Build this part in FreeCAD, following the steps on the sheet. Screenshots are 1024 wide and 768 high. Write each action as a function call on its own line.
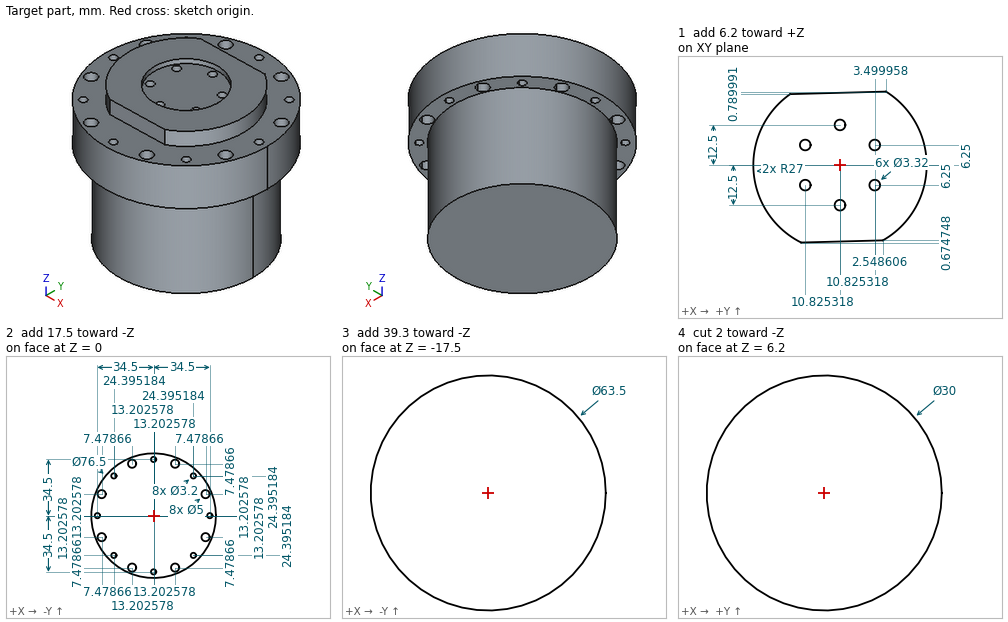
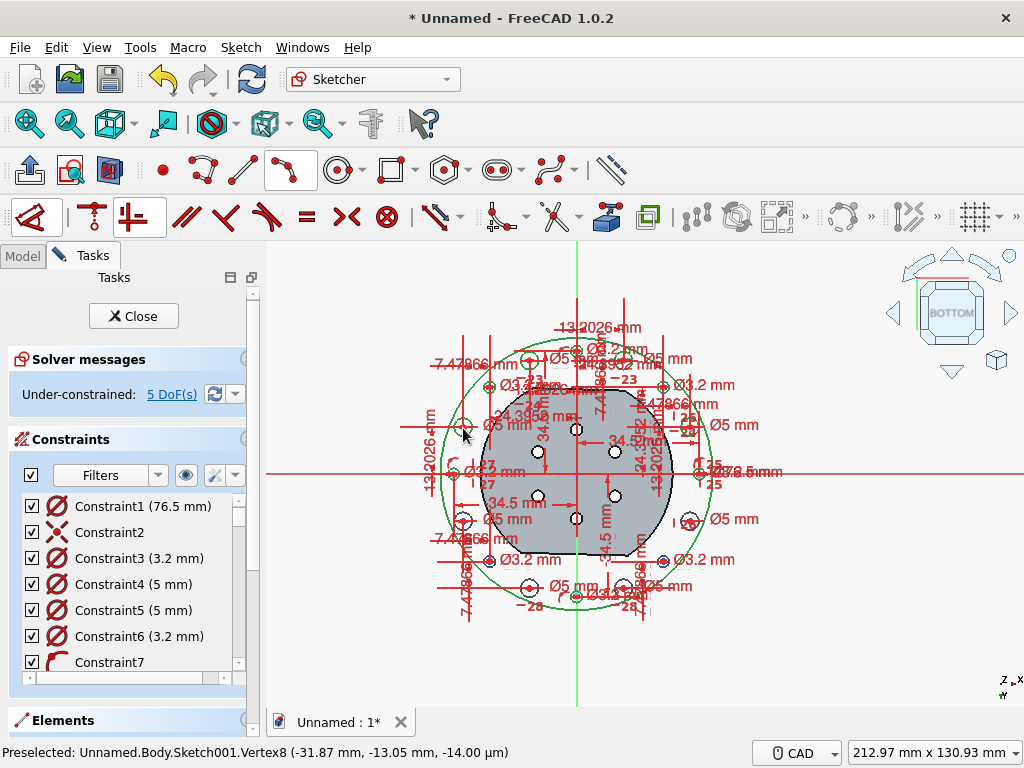
scroll(690, 521, up, 4)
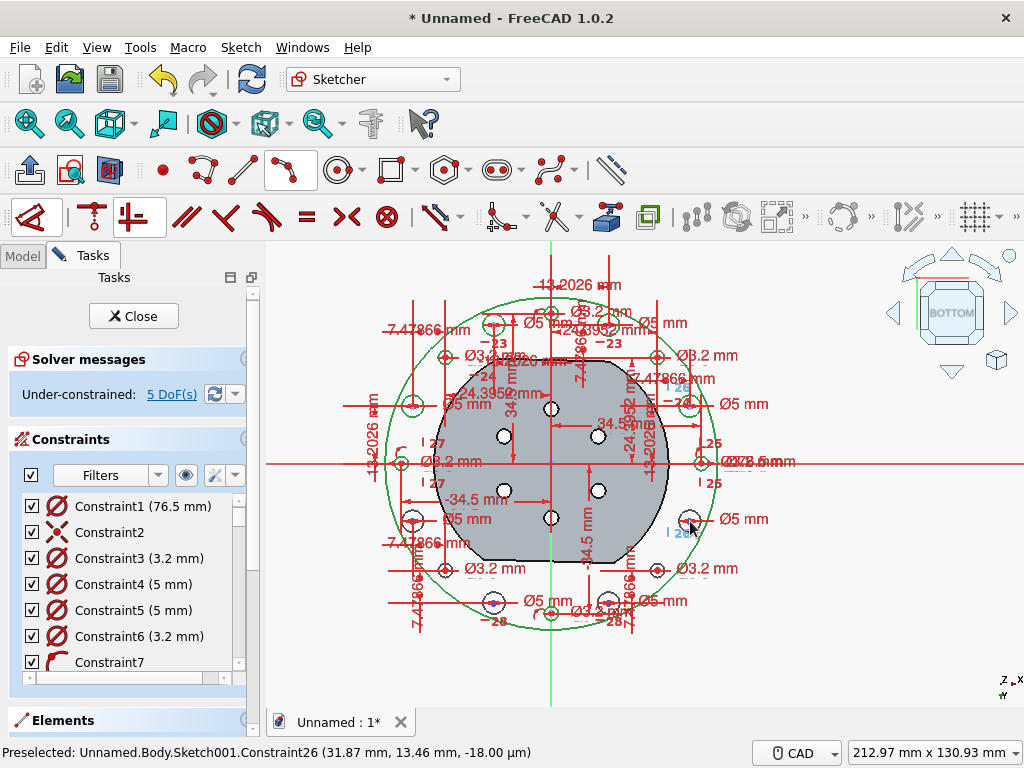
click(689, 521)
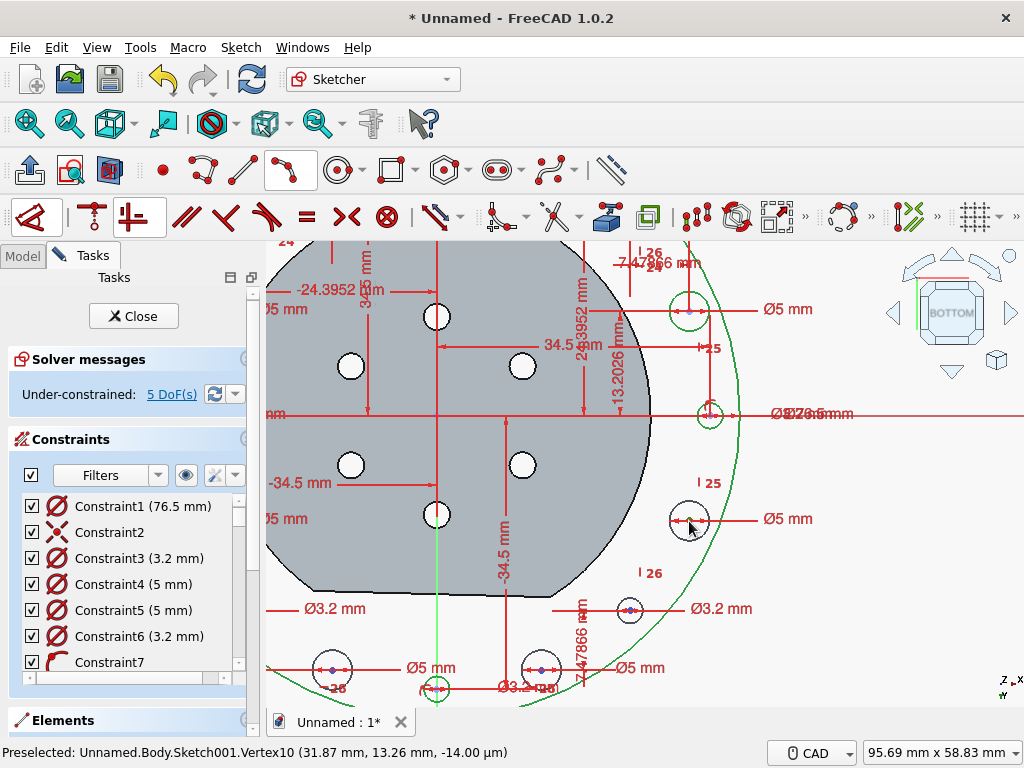
click(56, 218)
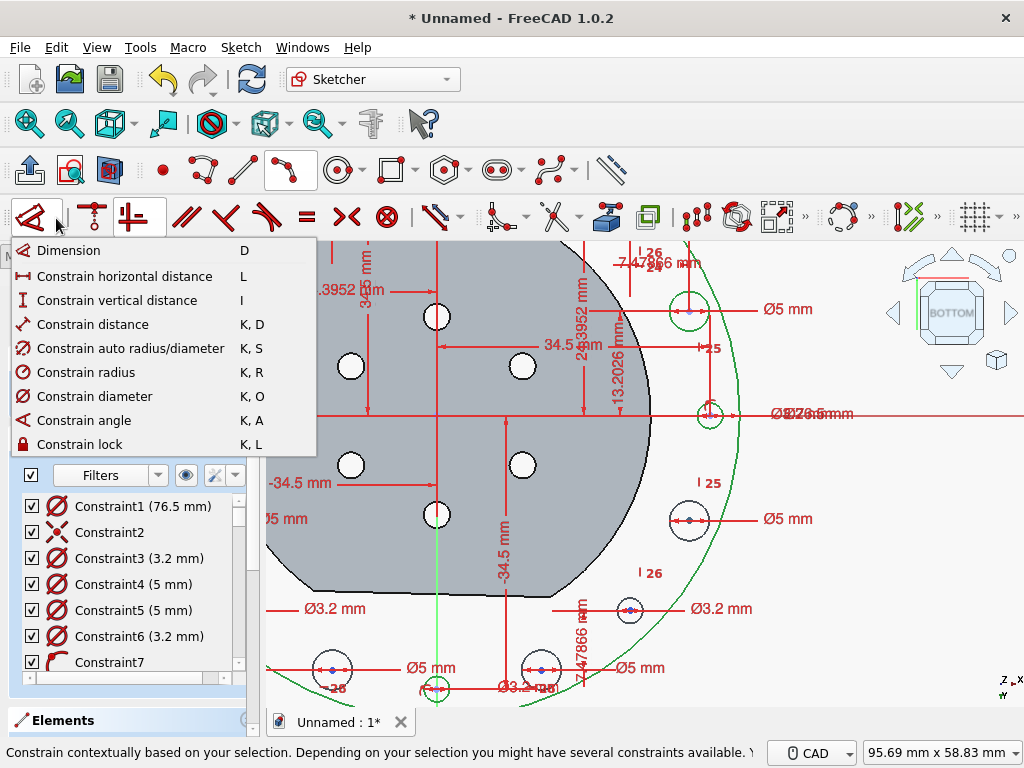
click(164, 300)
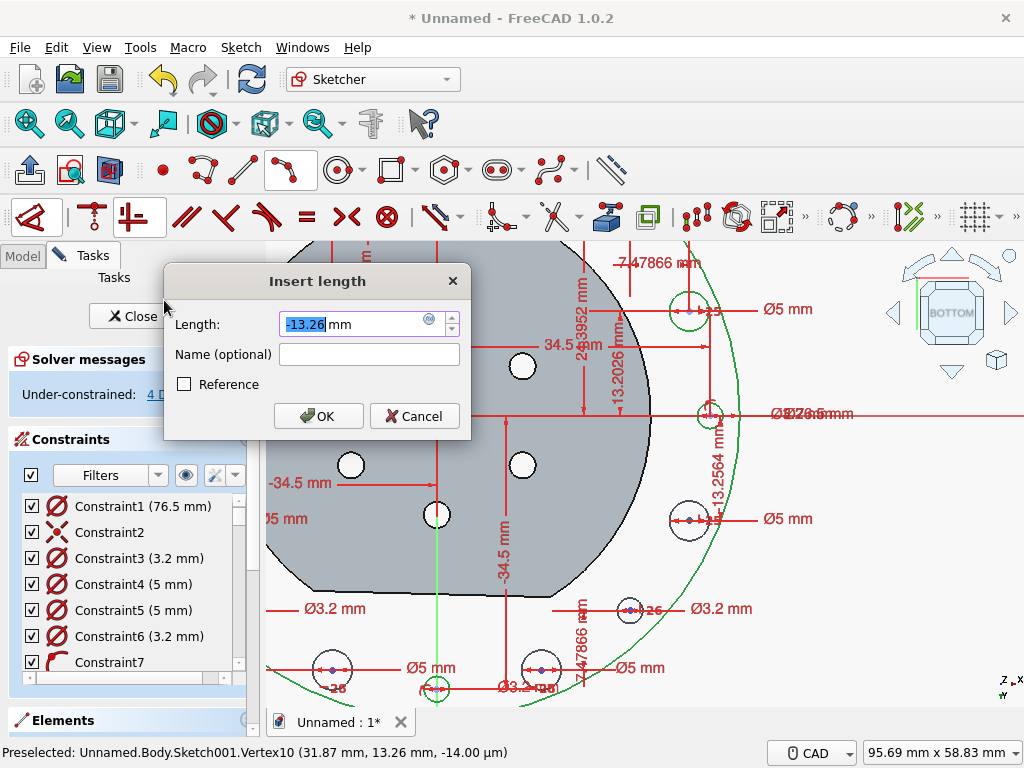
text(-13.202578)
key(Return)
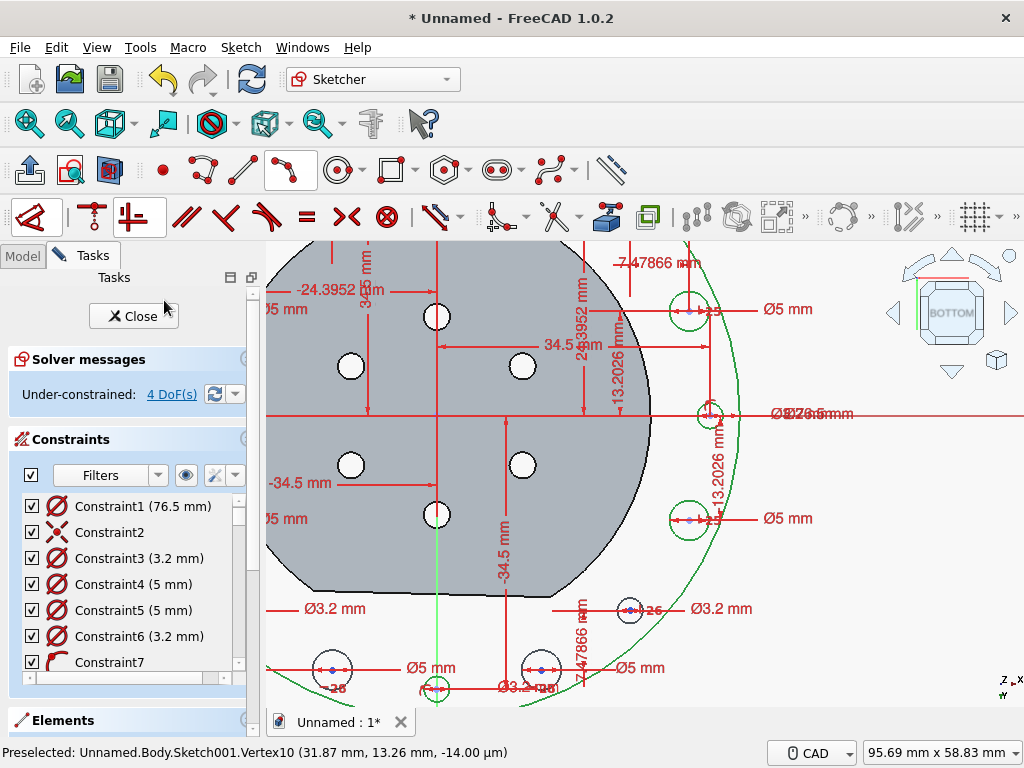
click(630, 611)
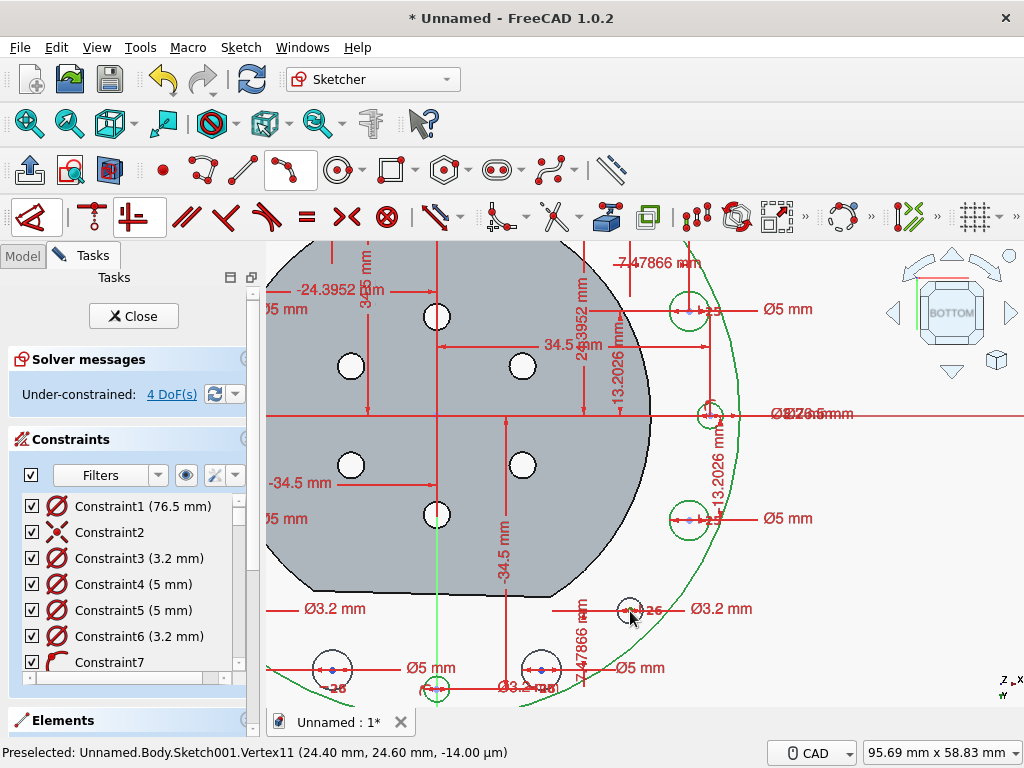
click(56, 218)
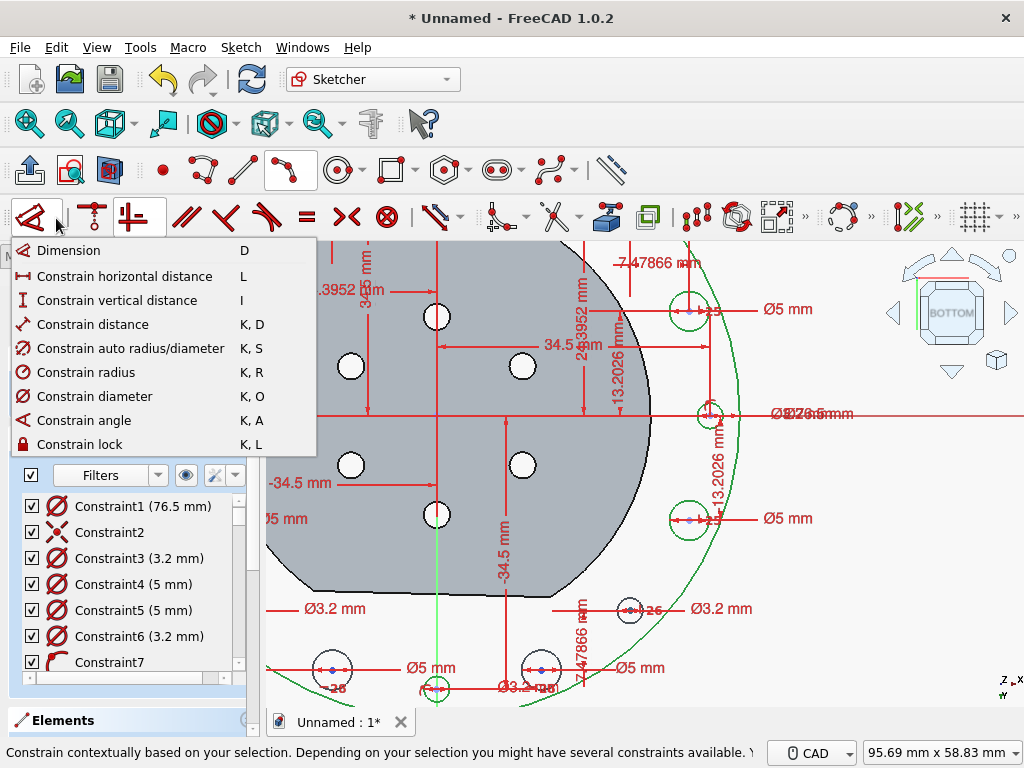
click(164, 300)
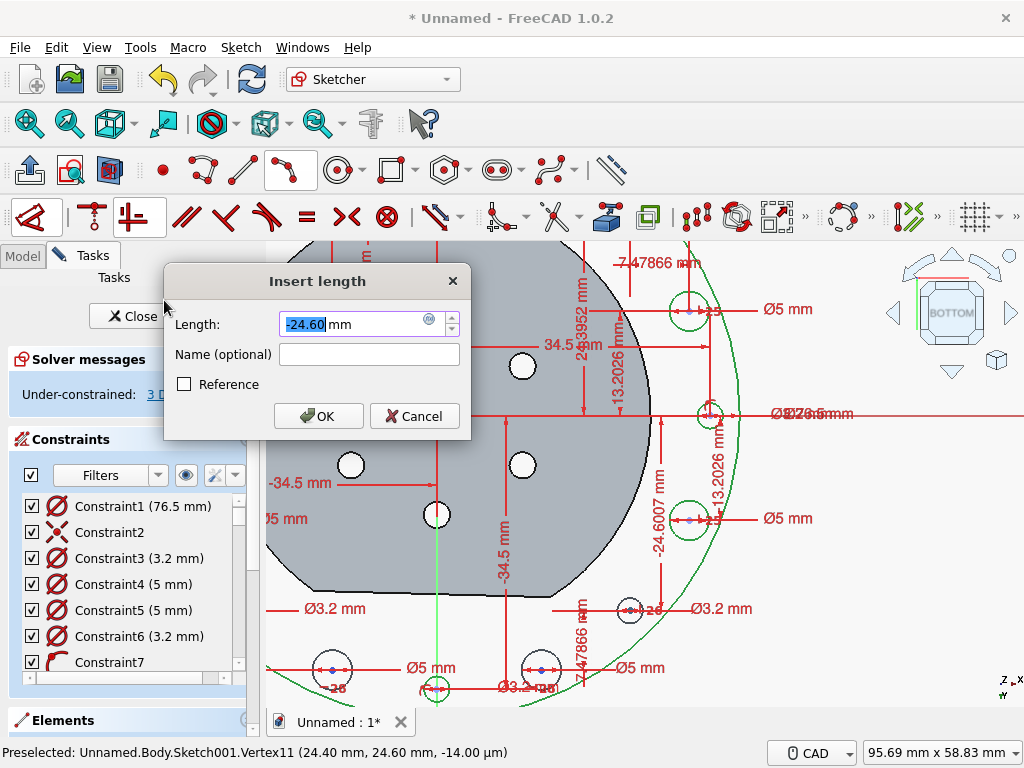
text(-24.395184)
key(Return)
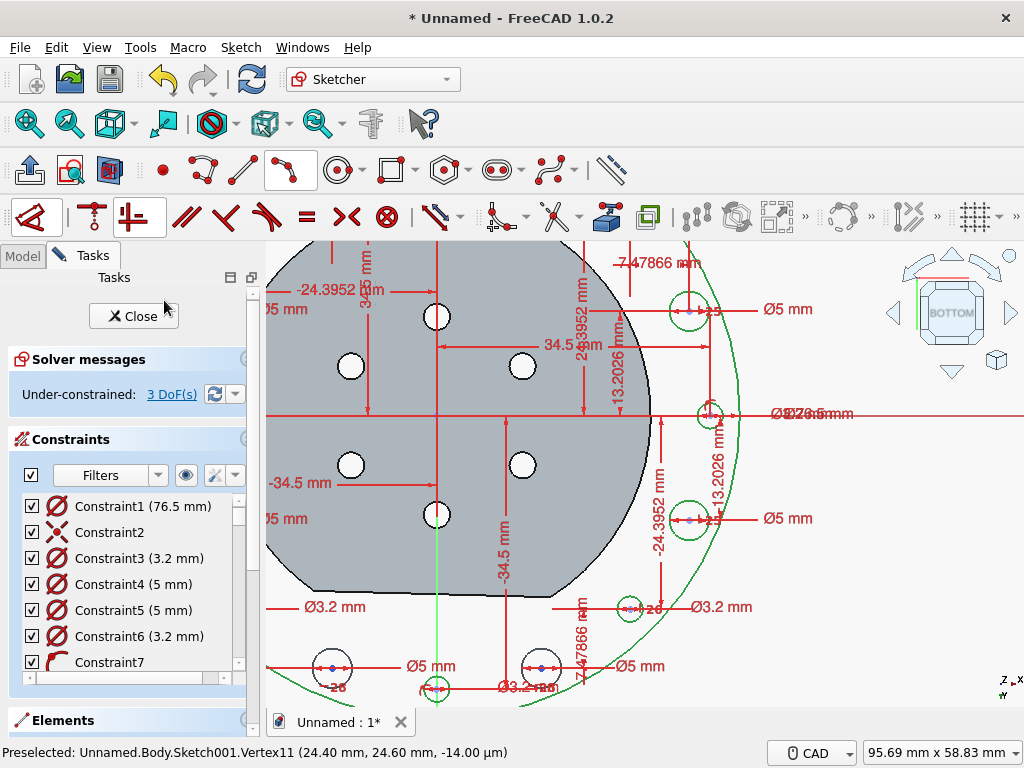
click(541, 668)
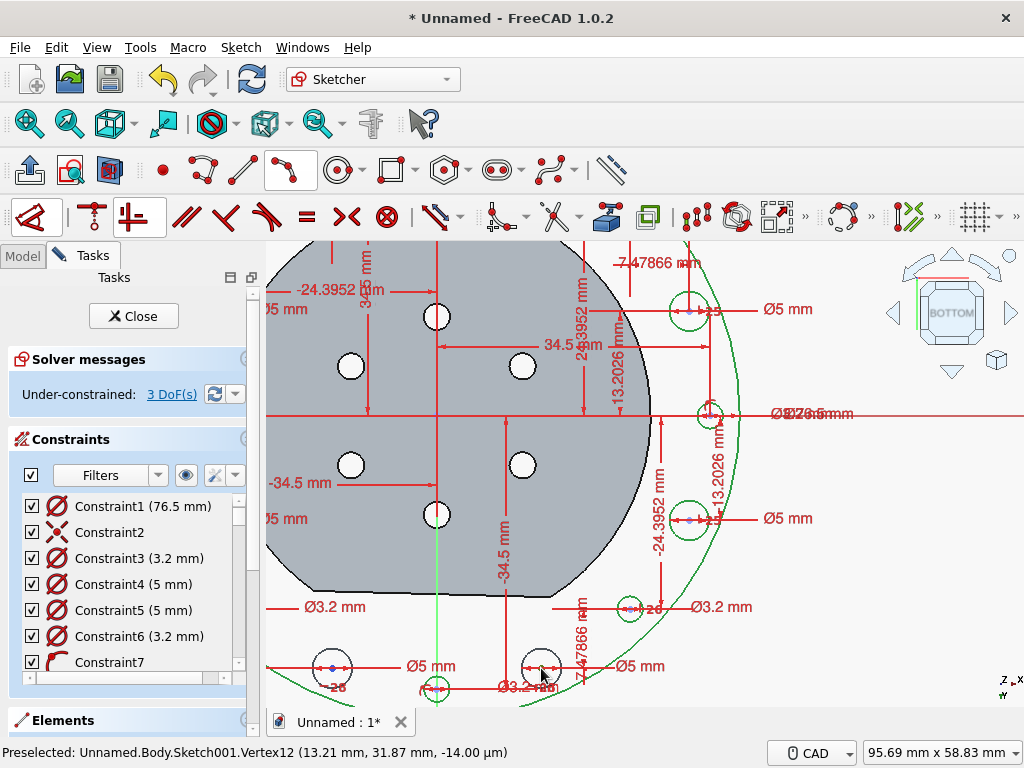
key(l)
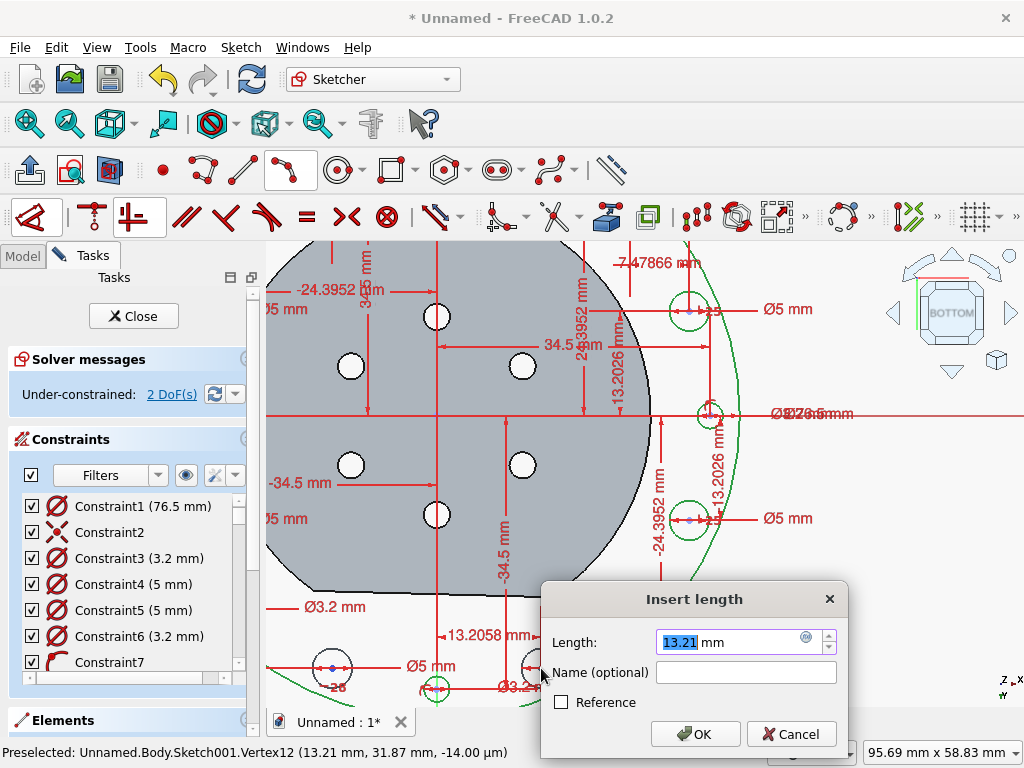
text(13.202578)
key(Return)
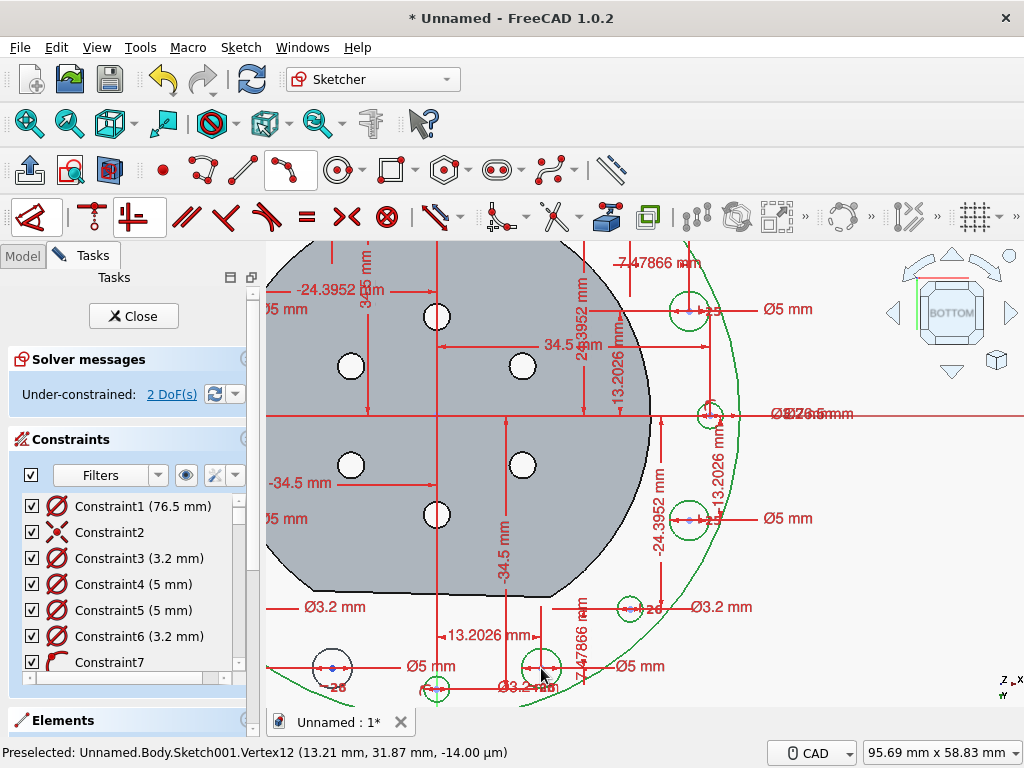
scroll(690, 521, down, 4)